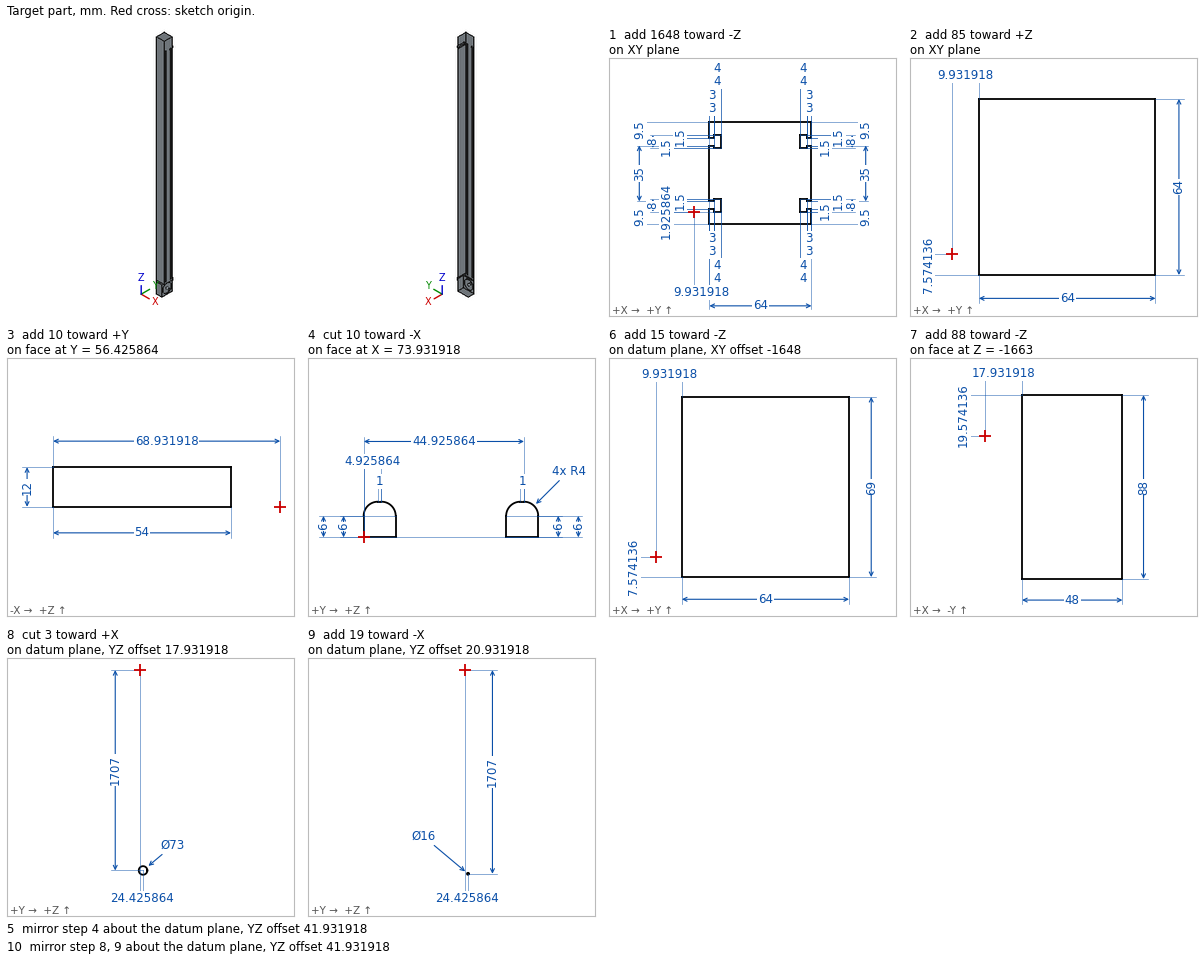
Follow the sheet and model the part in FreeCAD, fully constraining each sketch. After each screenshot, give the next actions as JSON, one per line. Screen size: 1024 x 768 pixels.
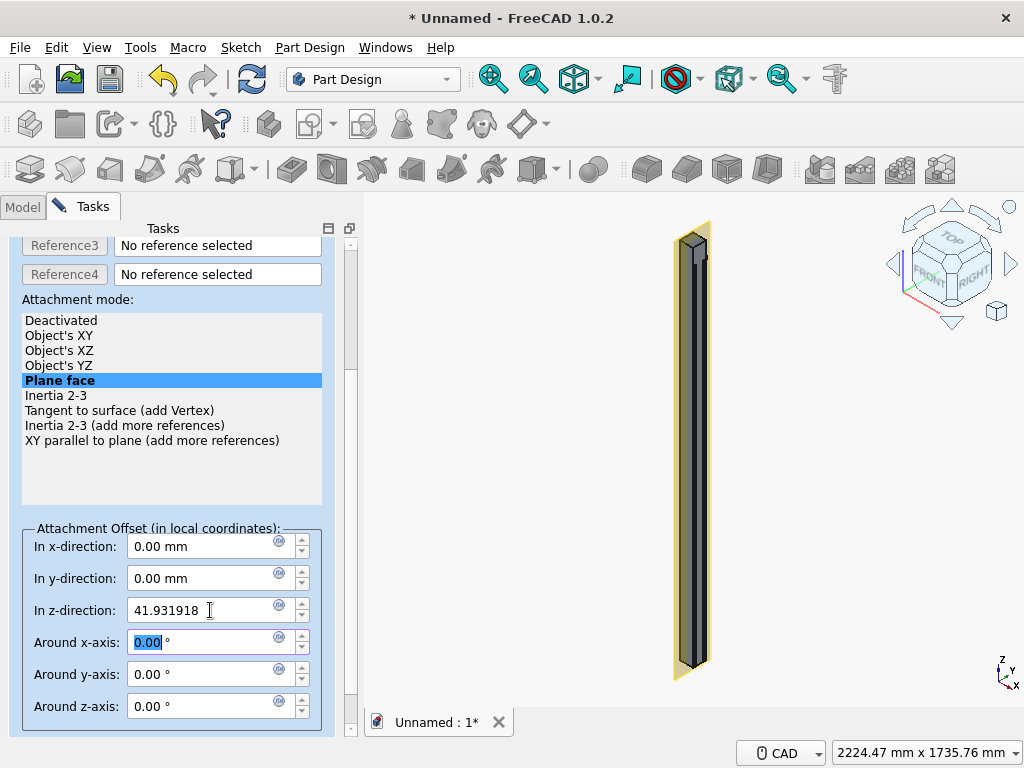
{"action": "scroll", "coordinate": [351, 487], "scroll_direction": "up", "scroll_amount": 4}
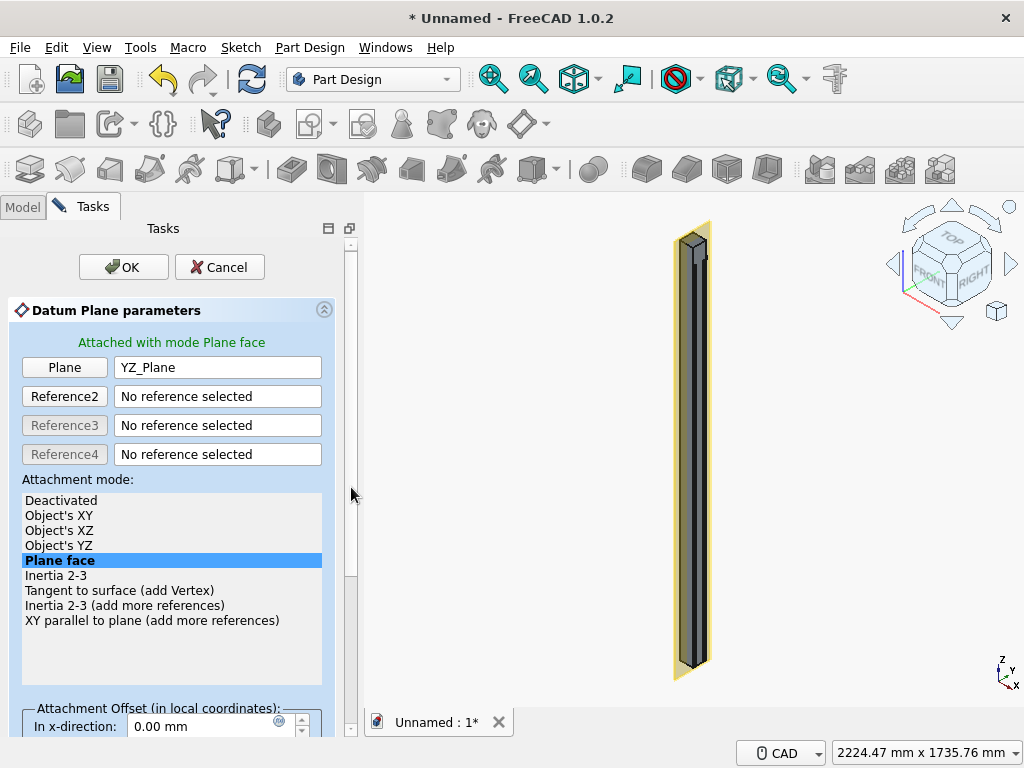
{"action": "left_click", "coordinate": [124, 267]}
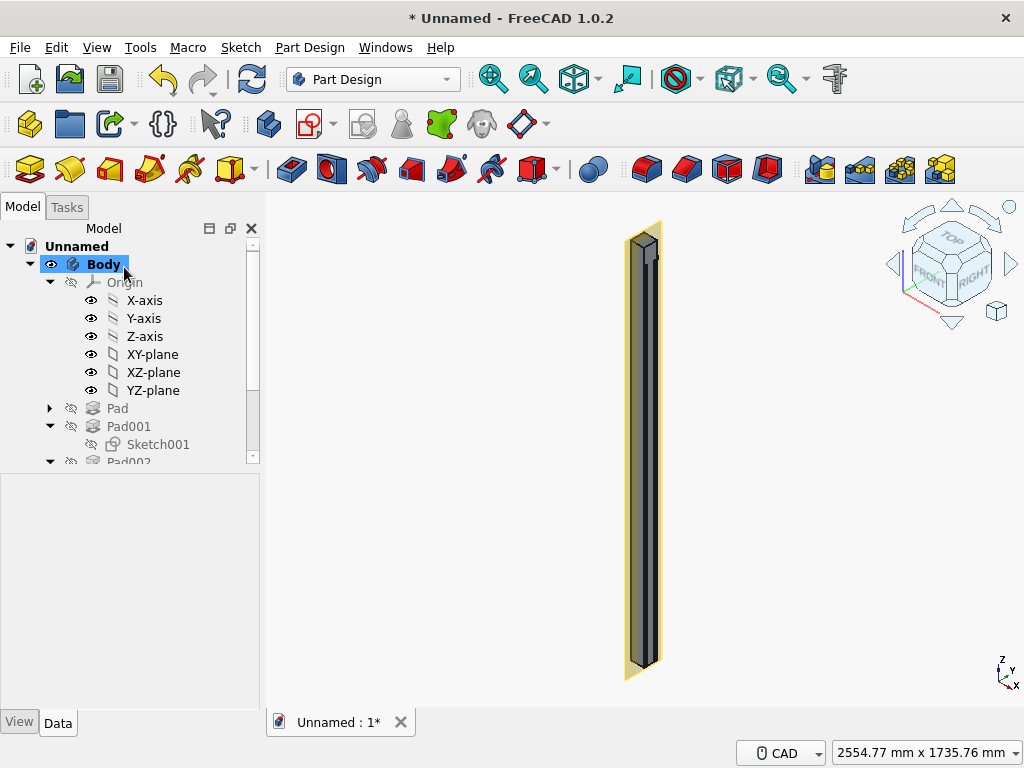
{"action": "scroll", "coordinate": [100, 350], "scroll_direction": "down", "scroll_amount": 3}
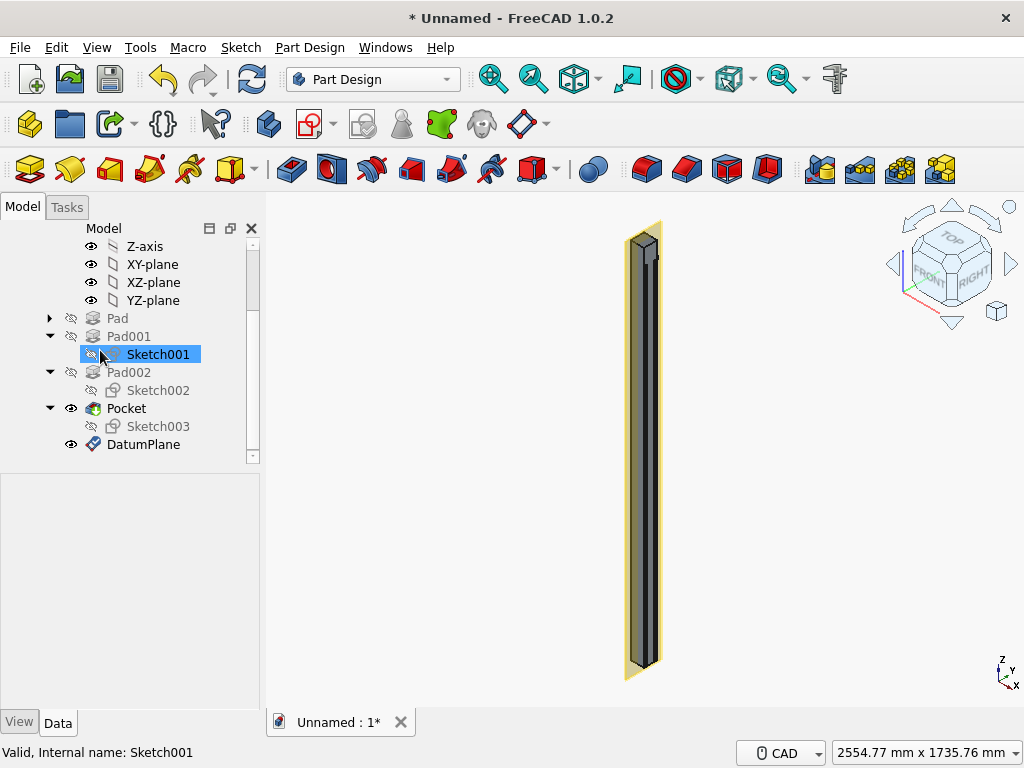
{"action": "left_click", "coordinate": [116, 408]}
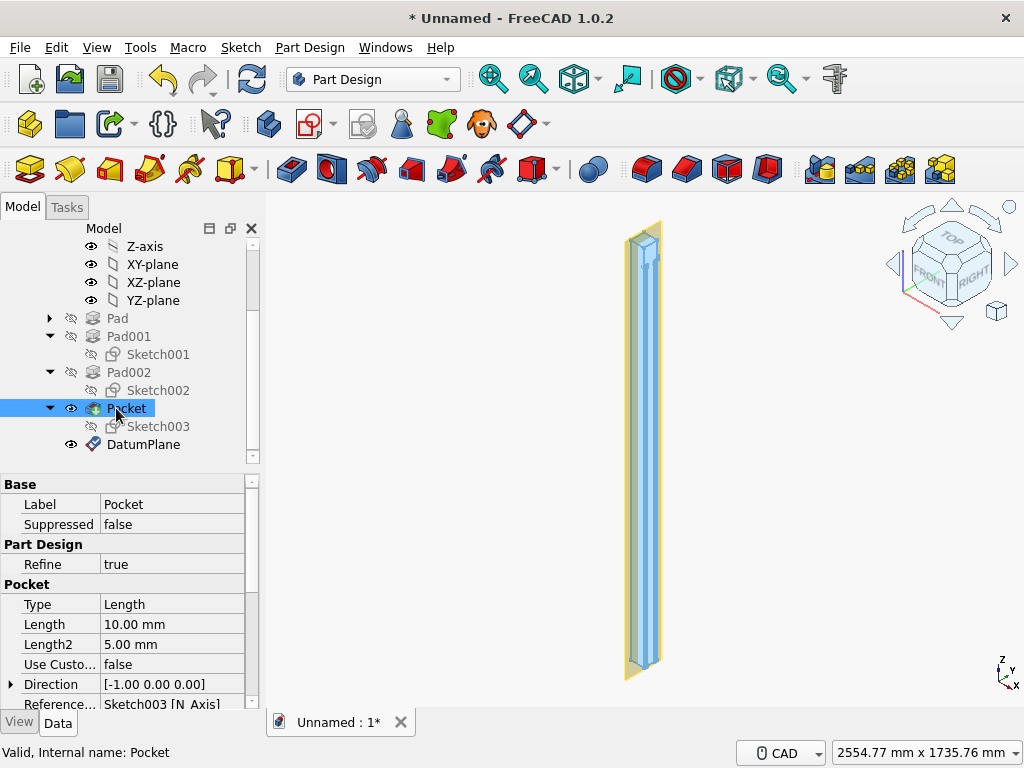
{"action": "left_click", "coordinate": [820, 170]}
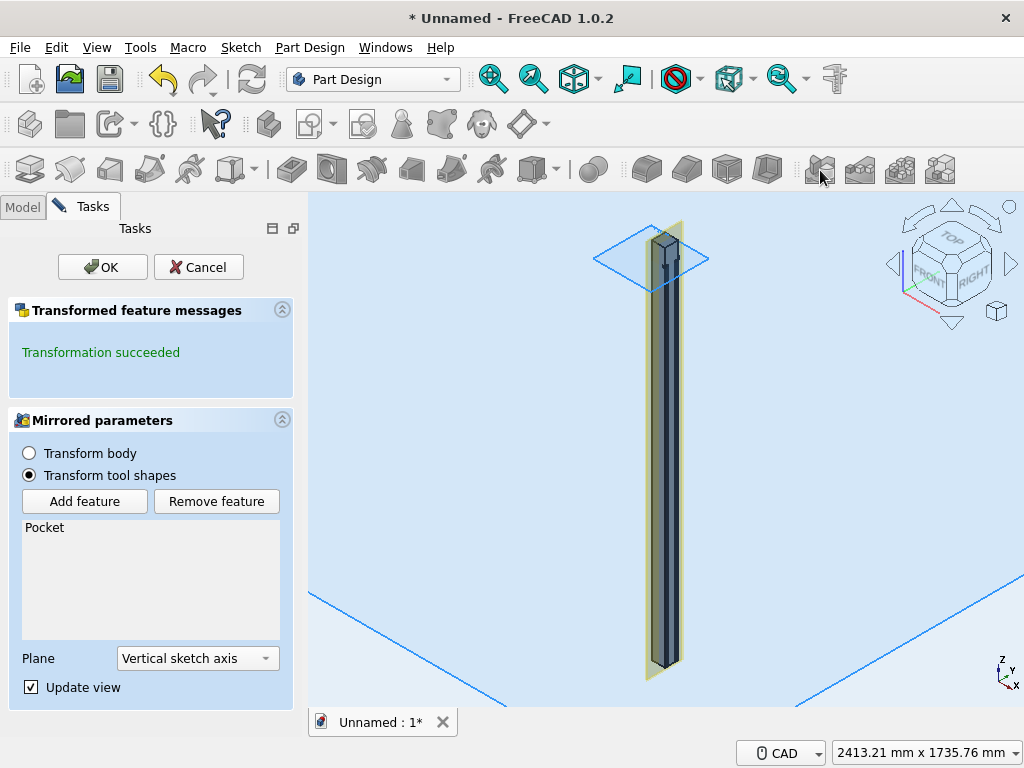
{"action": "left_click", "coordinate": [198, 658]}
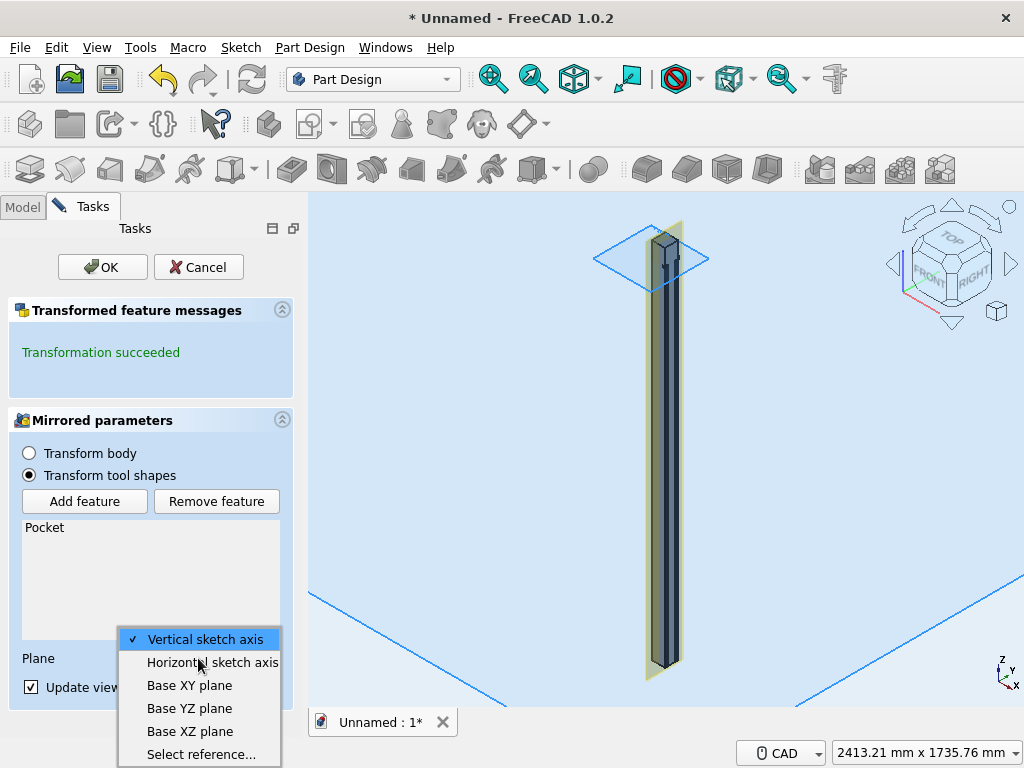
{"action": "left_click", "coordinate": [198, 754]}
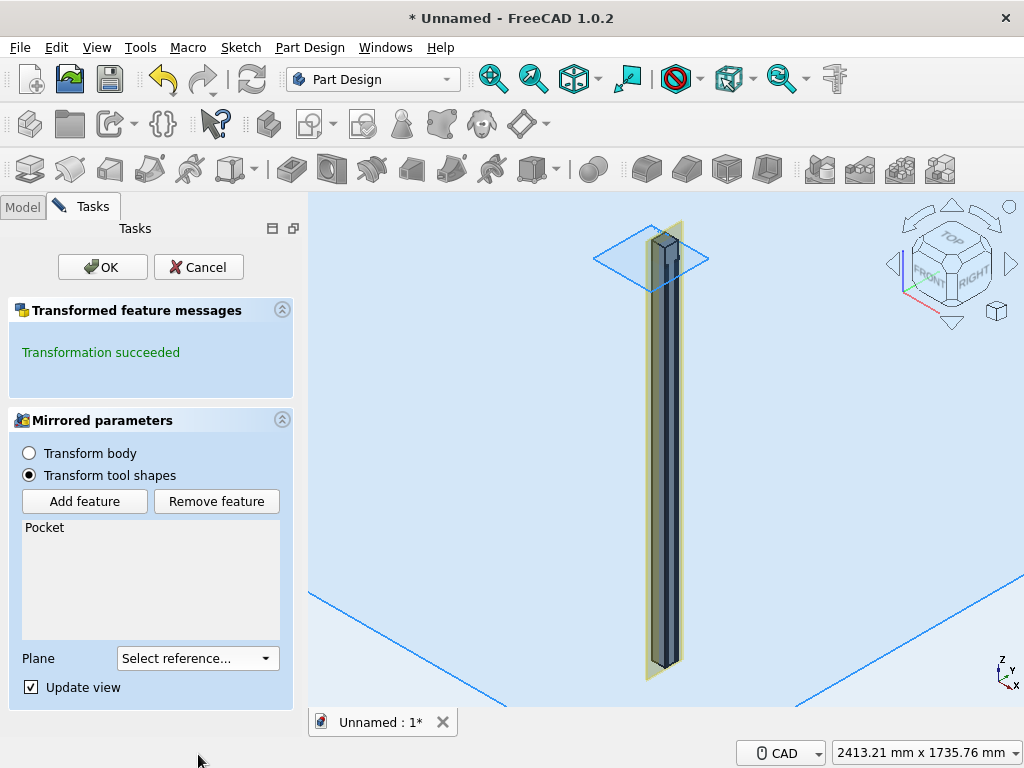
{"action": "left_click", "coordinate": [23, 206]}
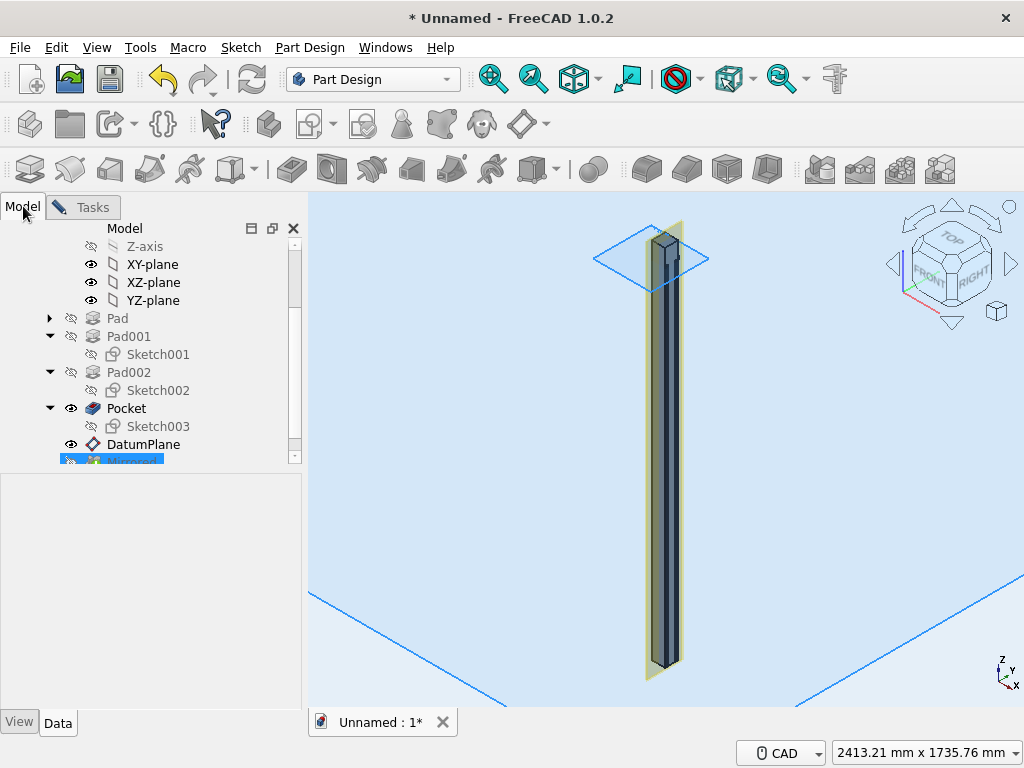
{"action": "left_click", "coordinate": [116, 444]}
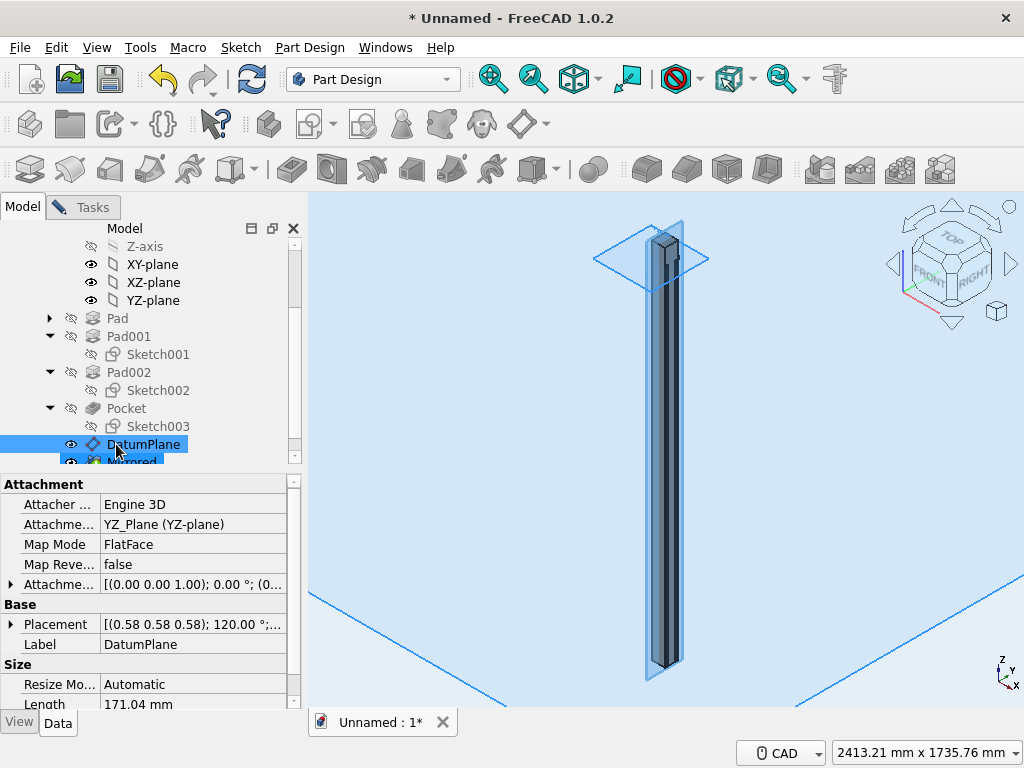
{"action": "left_click", "coordinate": [84, 206]}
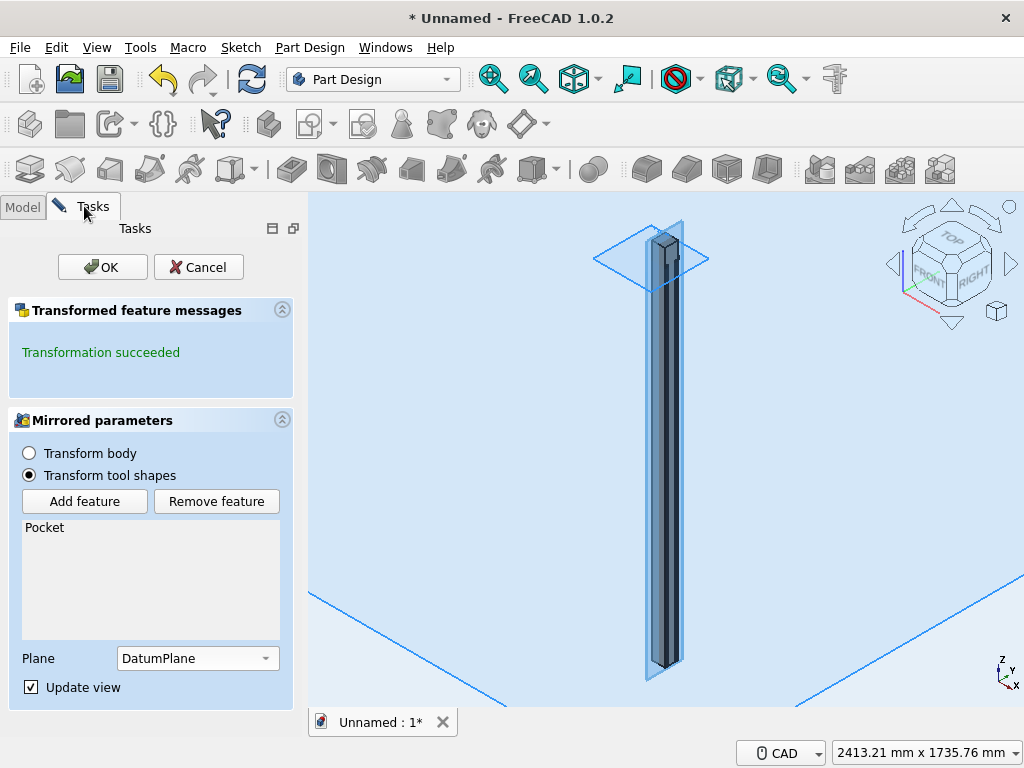
{"action": "left_click", "coordinate": [103, 267]}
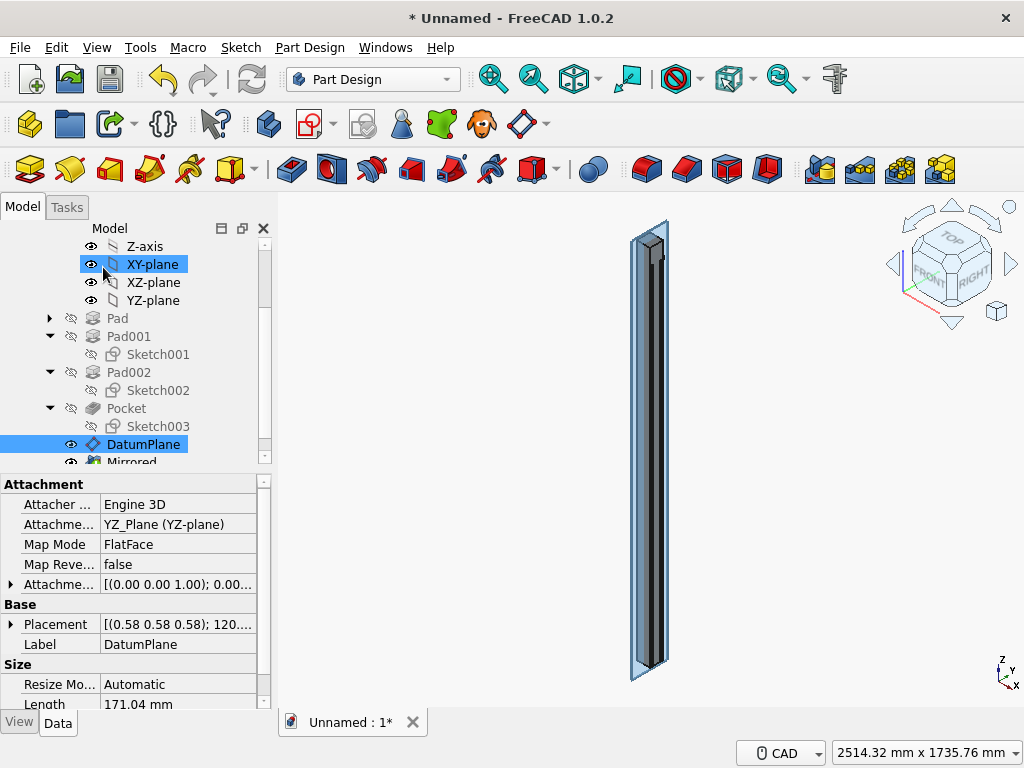
{"action": "left_click", "coordinate": [116, 444]}
{"action": "key", "text": "space"}